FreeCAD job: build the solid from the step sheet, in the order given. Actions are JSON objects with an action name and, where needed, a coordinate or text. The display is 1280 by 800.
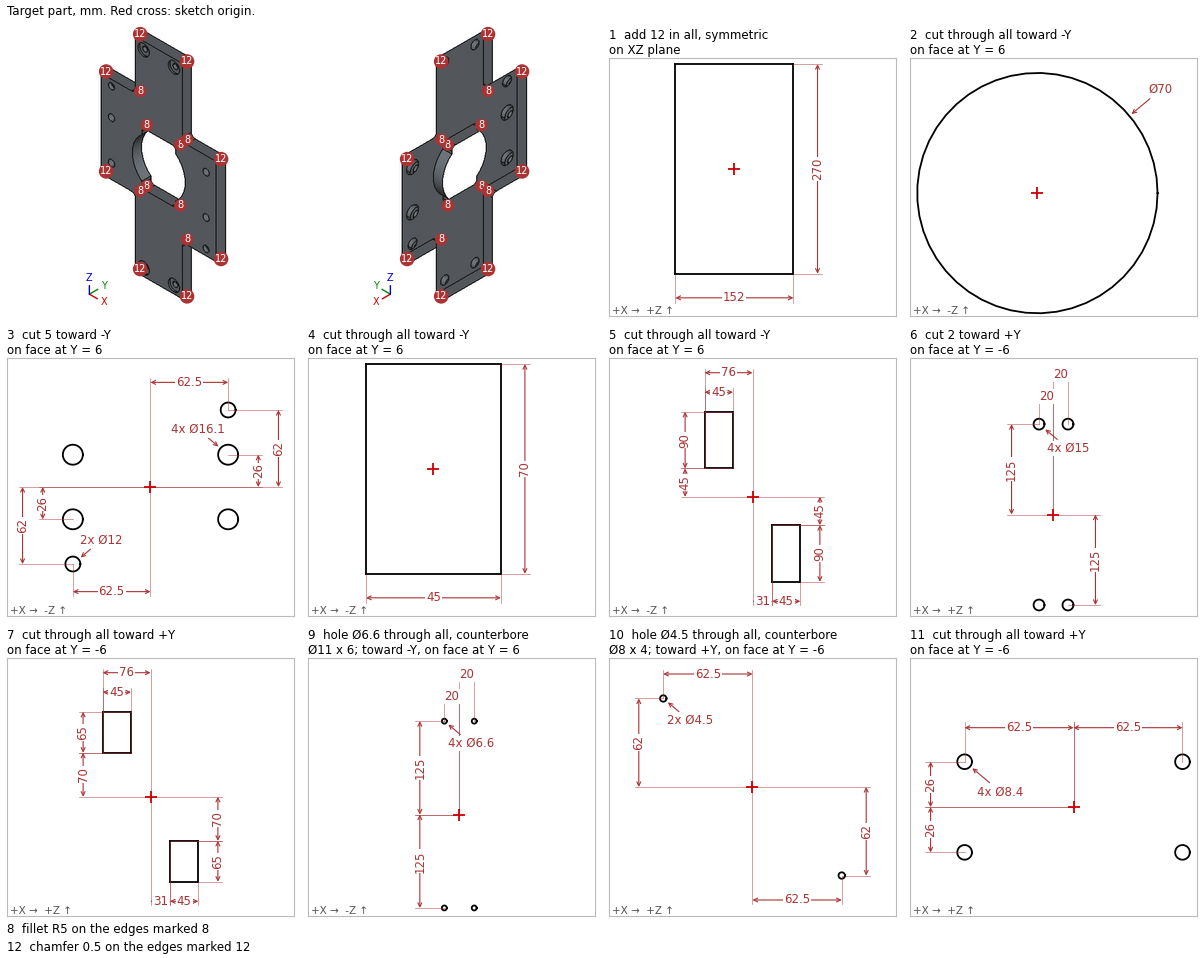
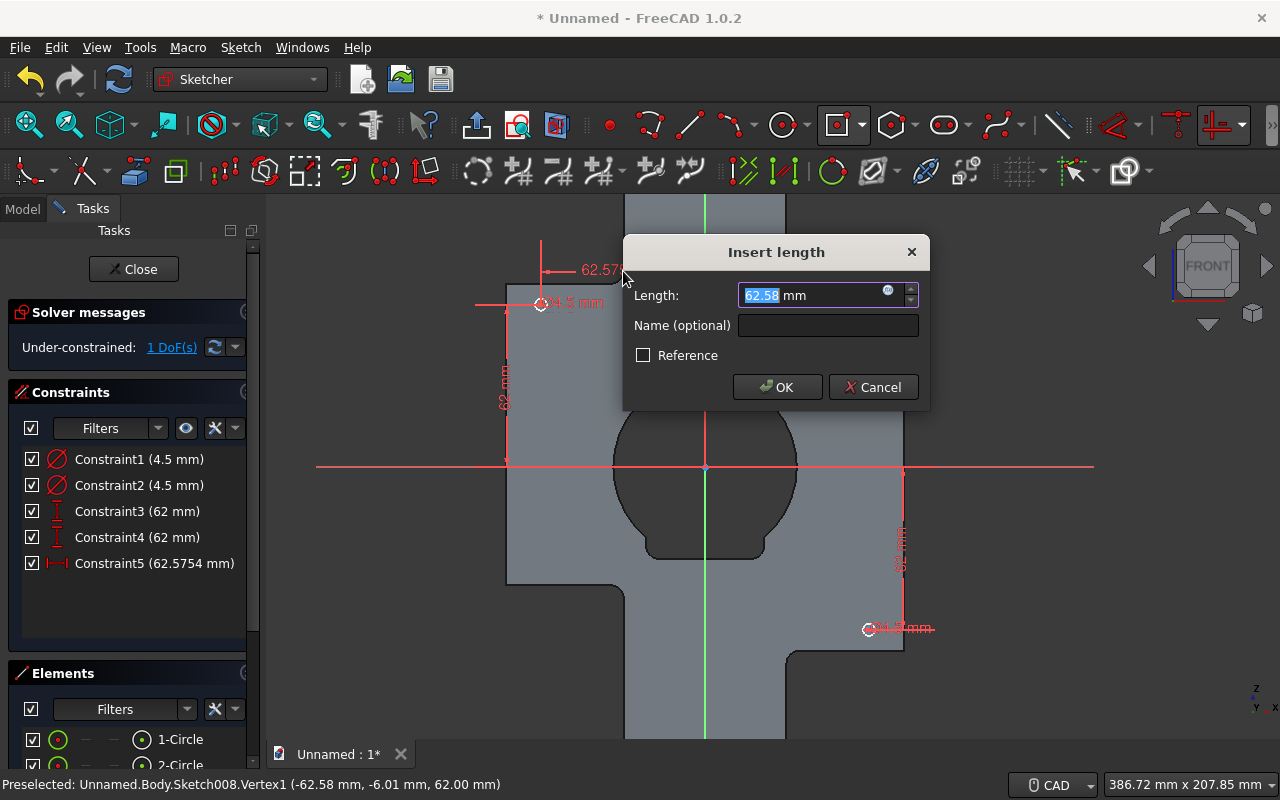
{"action": "type", "text": "62.5"}
{"action": "key", "text": "Return"}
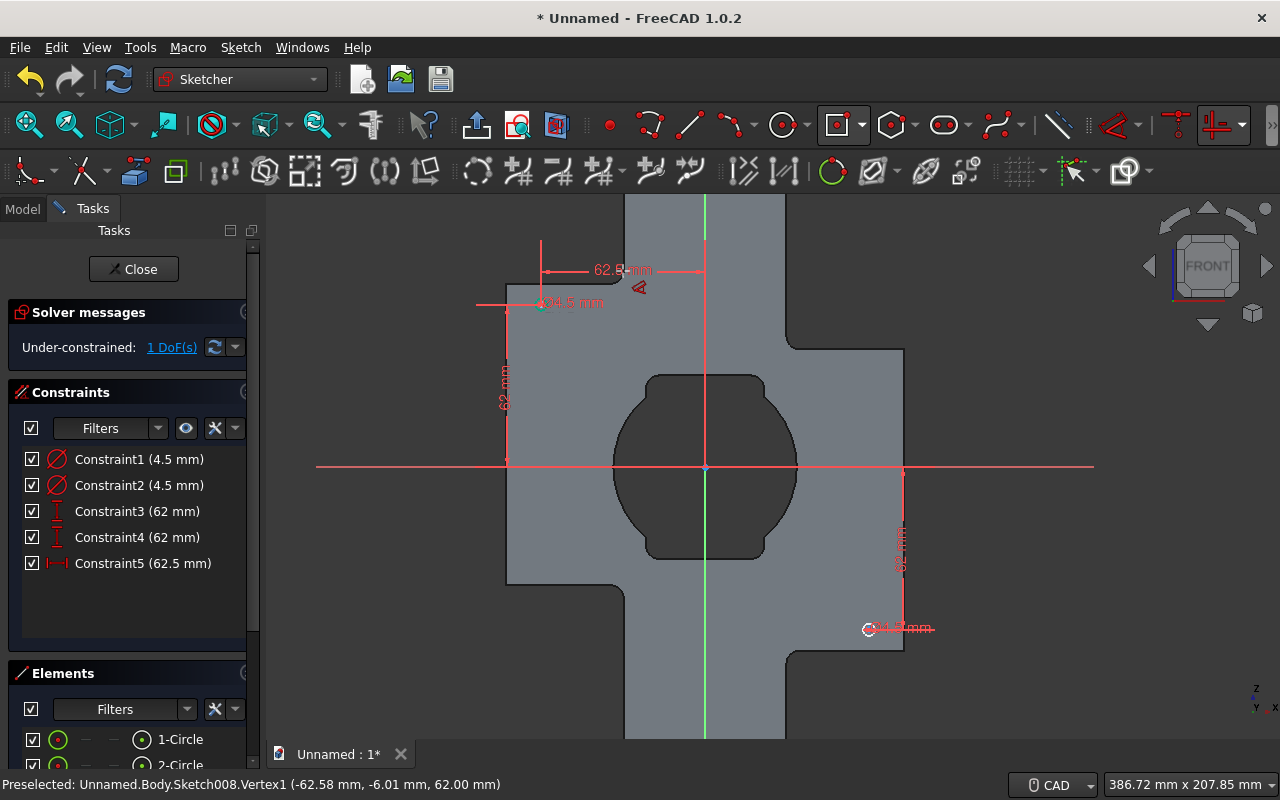
{"action": "left_click", "coordinate": [869, 630]}
{"action": "left_click", "coordinate": [787, 664]}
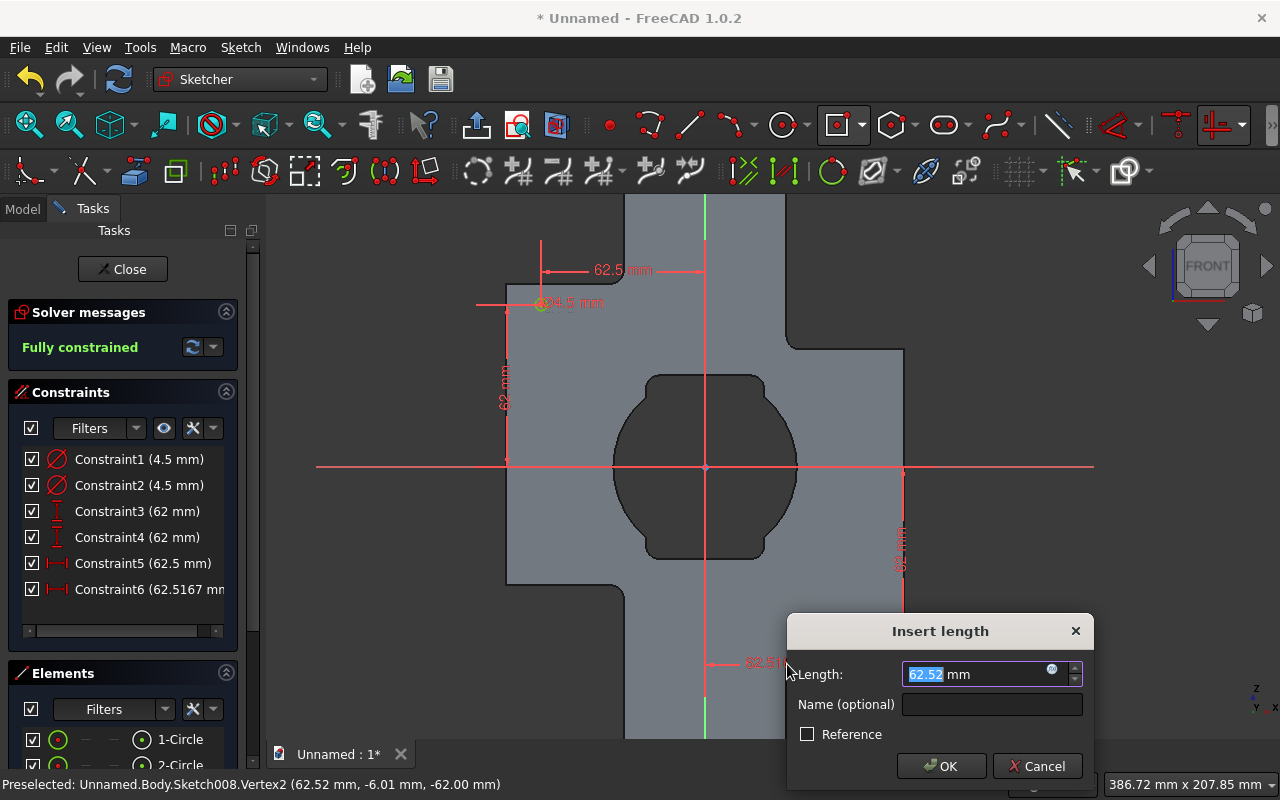
{"action": "type", "text": "62.5"}
{"action": "key", "text": "Return"}
{"action": "key", "text": "Escape"}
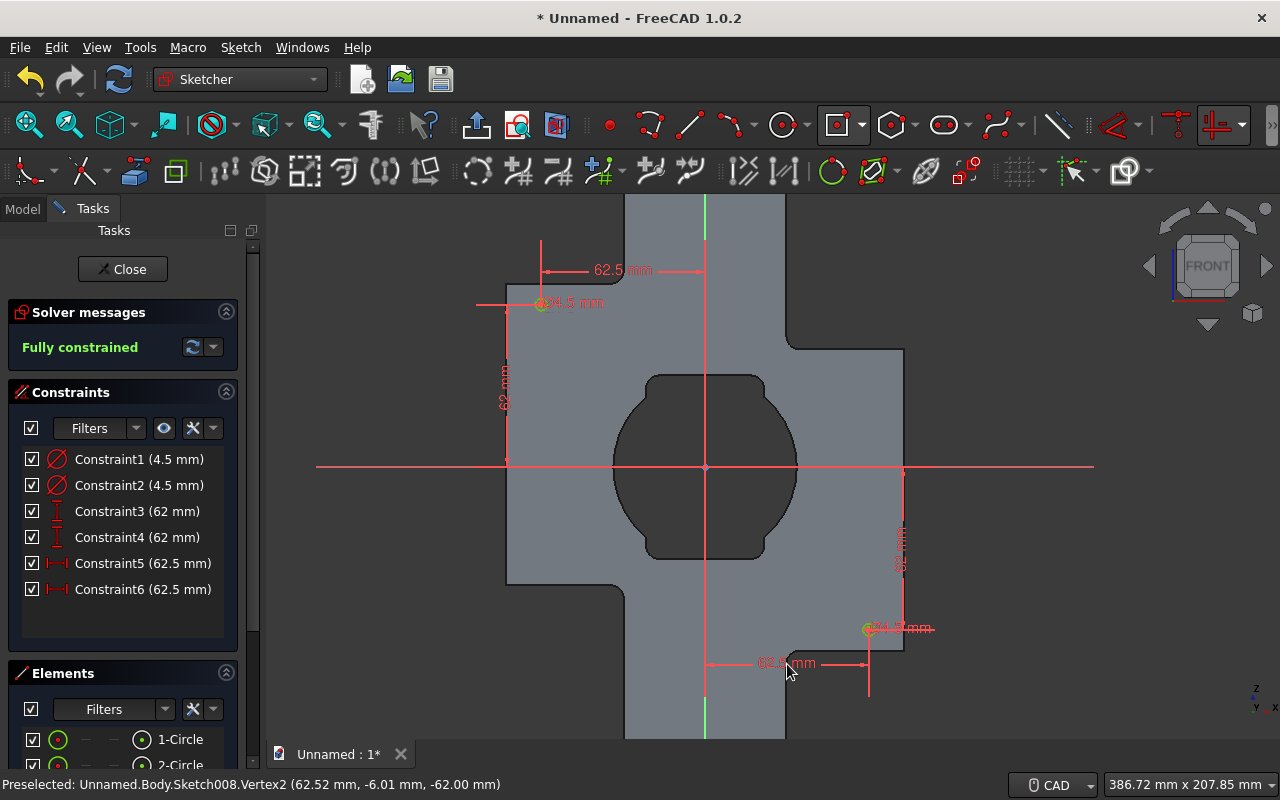
{"action": "left_click", "coordinate": [123, 269]}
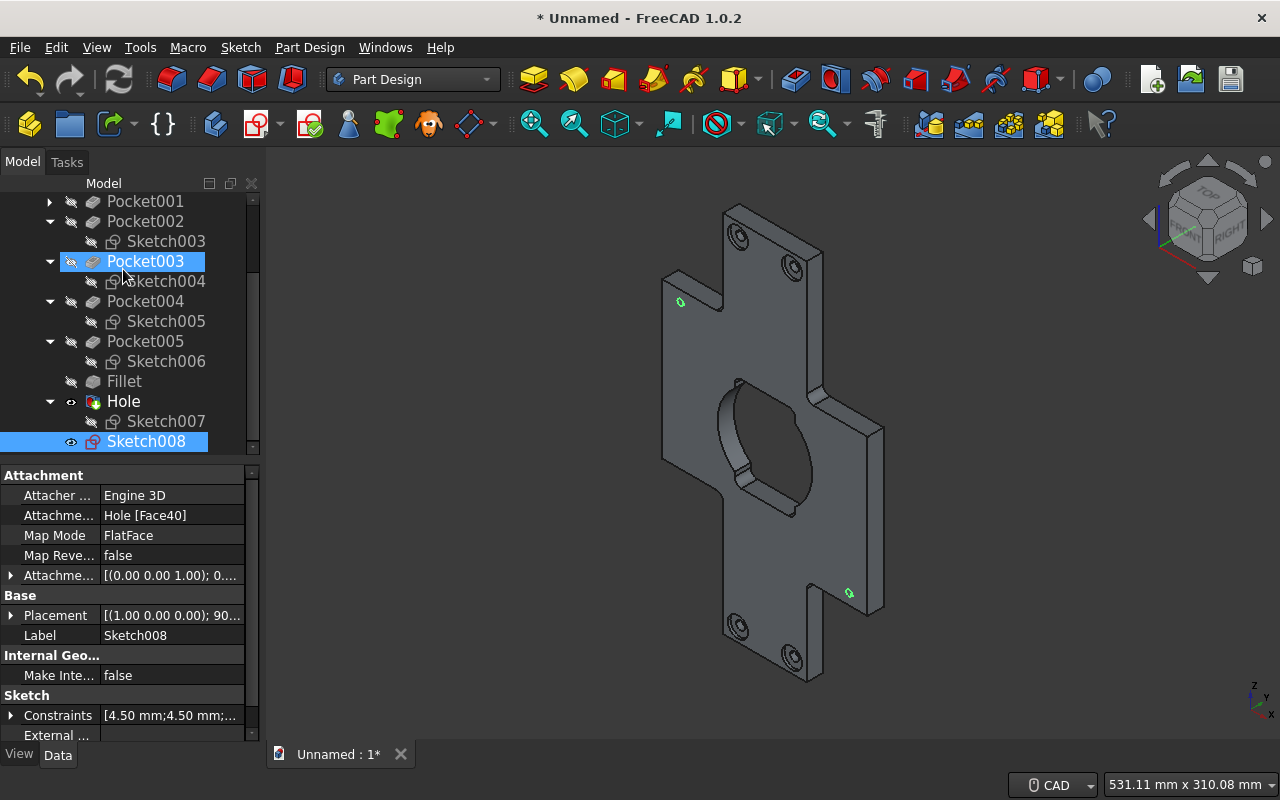
{"action": "left_click", "coordinate": [836, 80]}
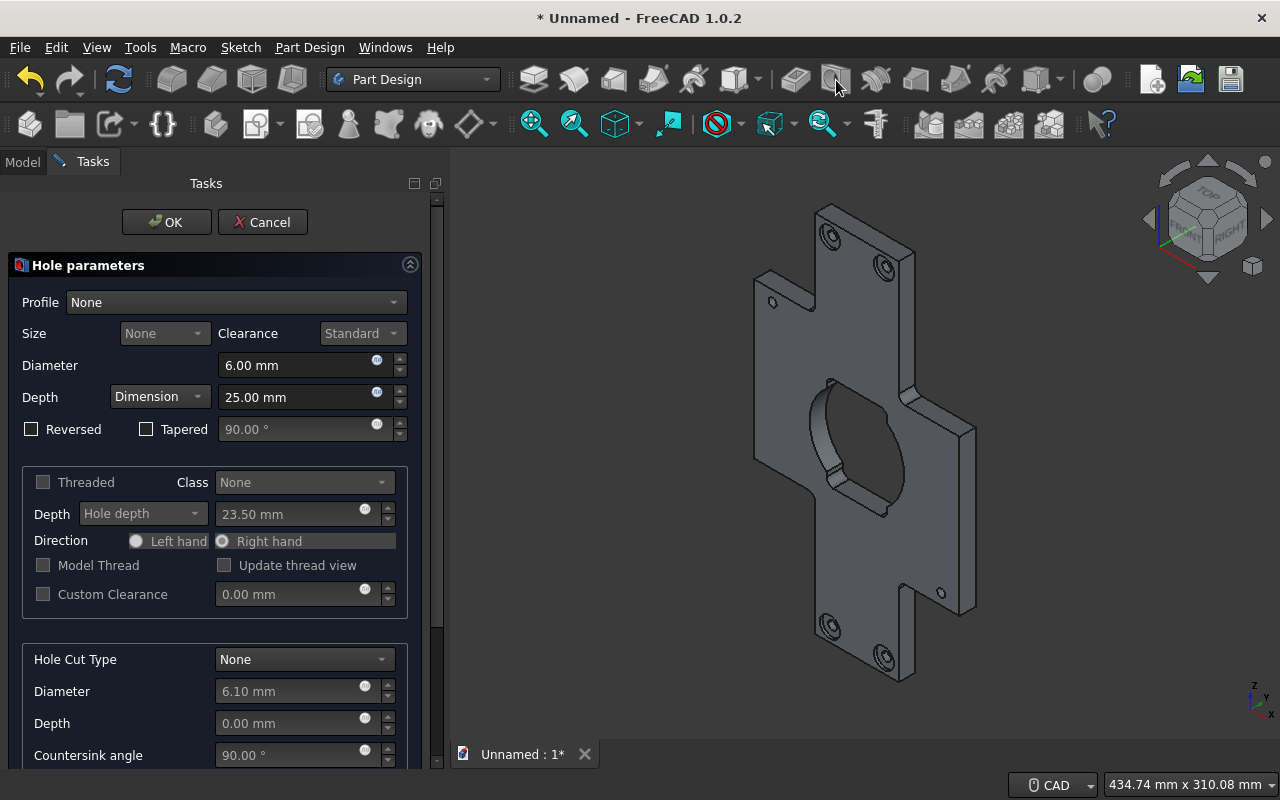
{"action": "triple_click", "coordinate": [305, 365]}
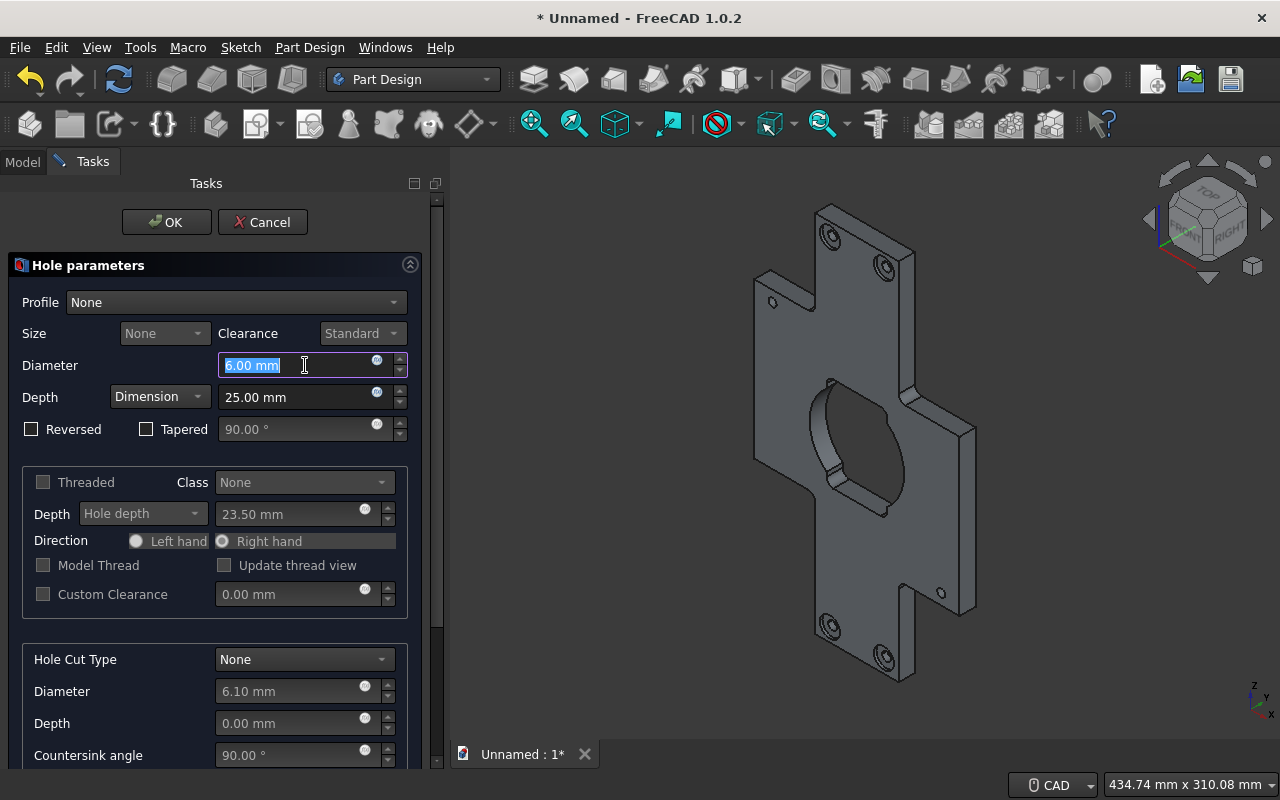
{"action": "type", "text": "4.5"}
{"action": "key", "text": "Tab"}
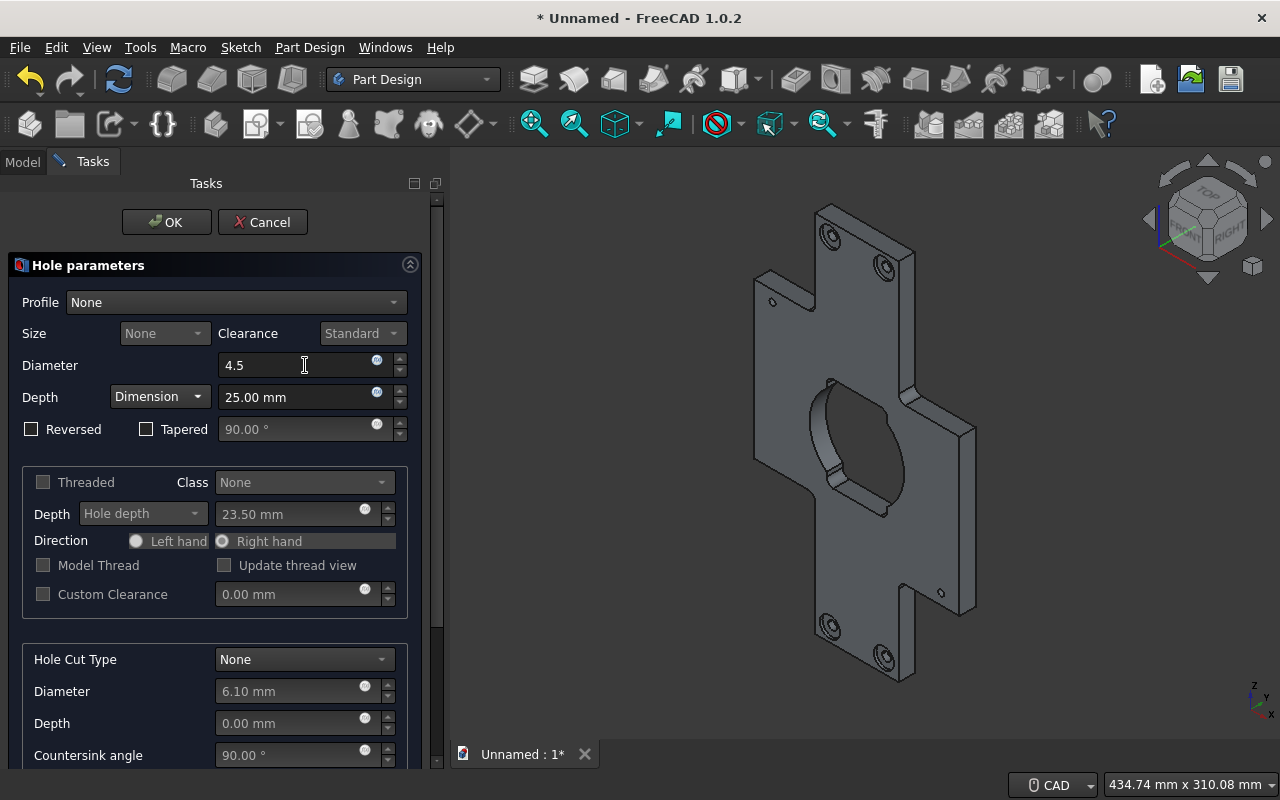
{"action": "left_click", "coordinate": [161, 396]}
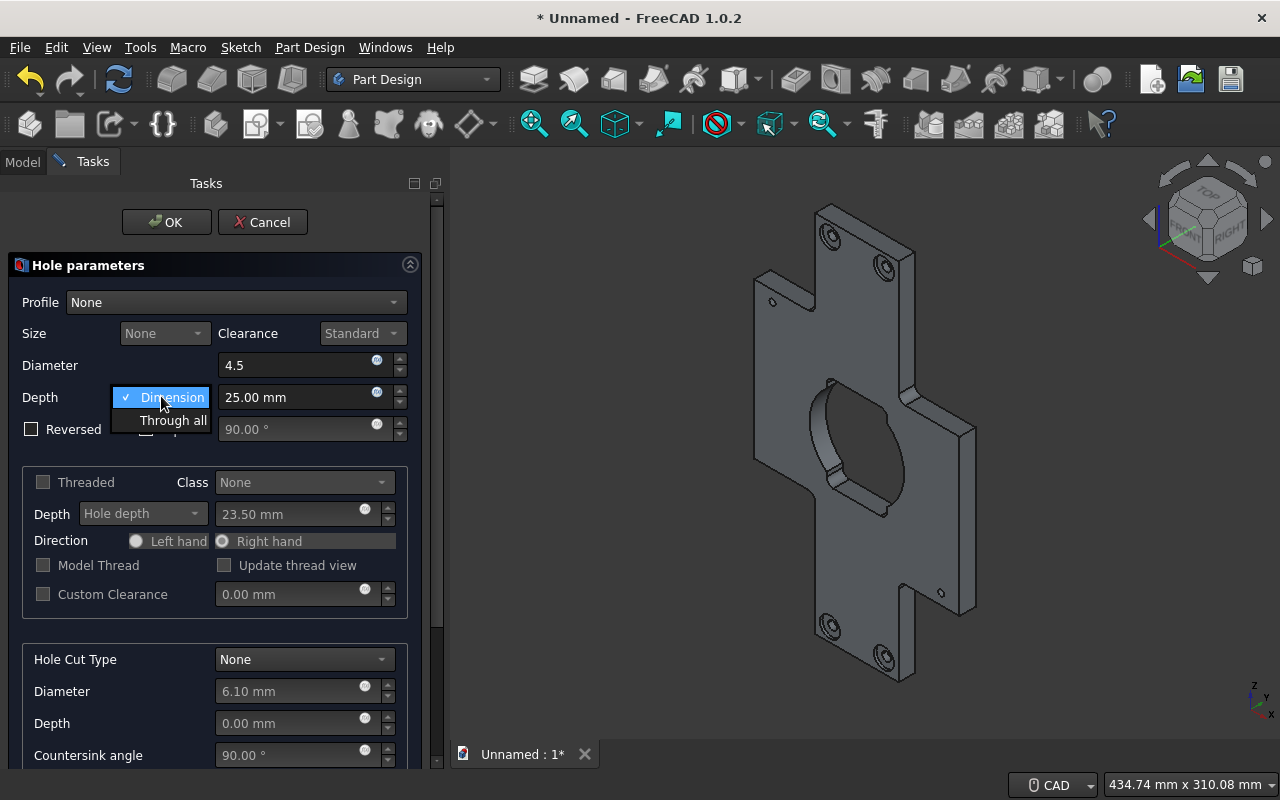
{"action": "left_click", "coordinate": [160, 420]}